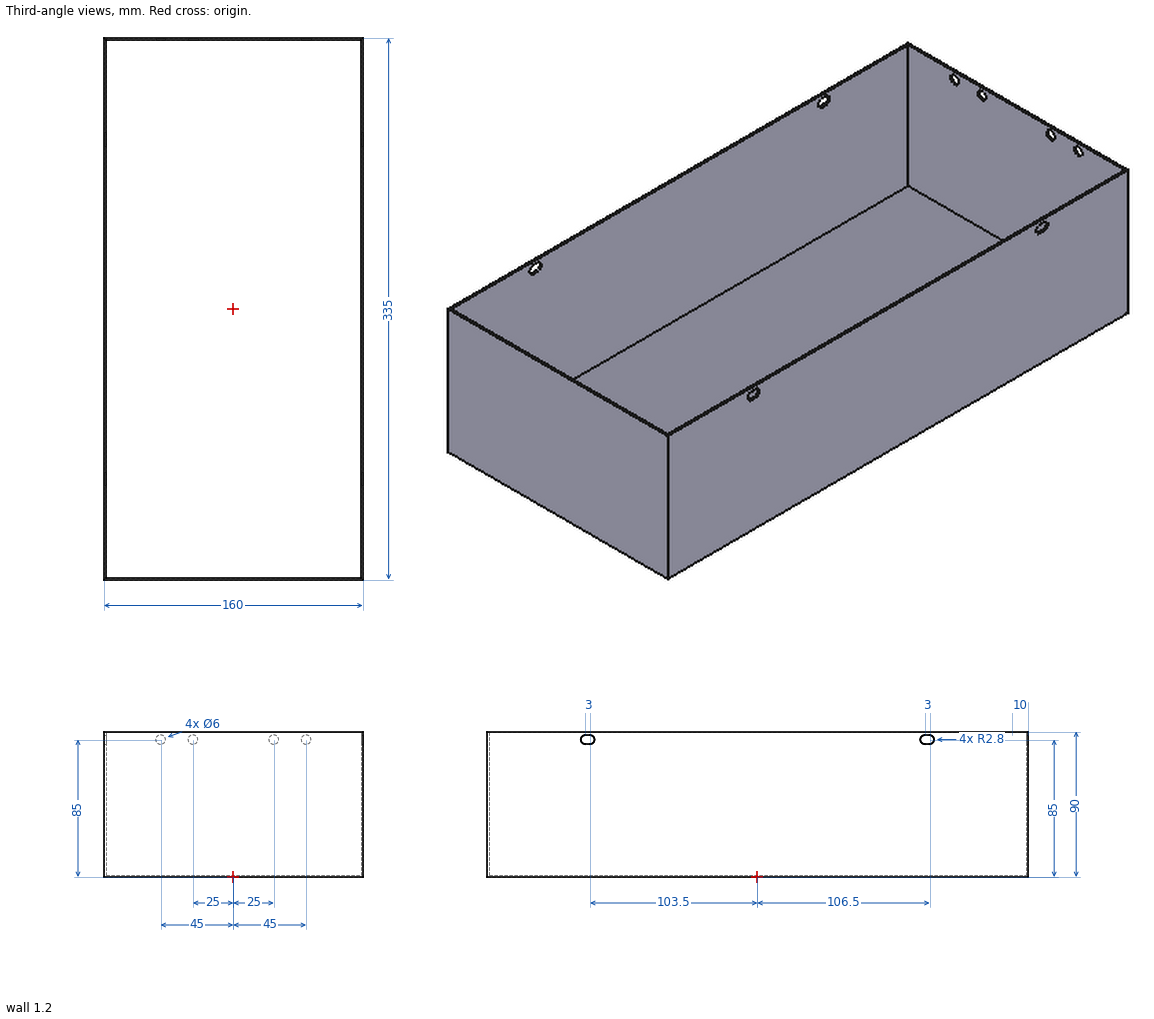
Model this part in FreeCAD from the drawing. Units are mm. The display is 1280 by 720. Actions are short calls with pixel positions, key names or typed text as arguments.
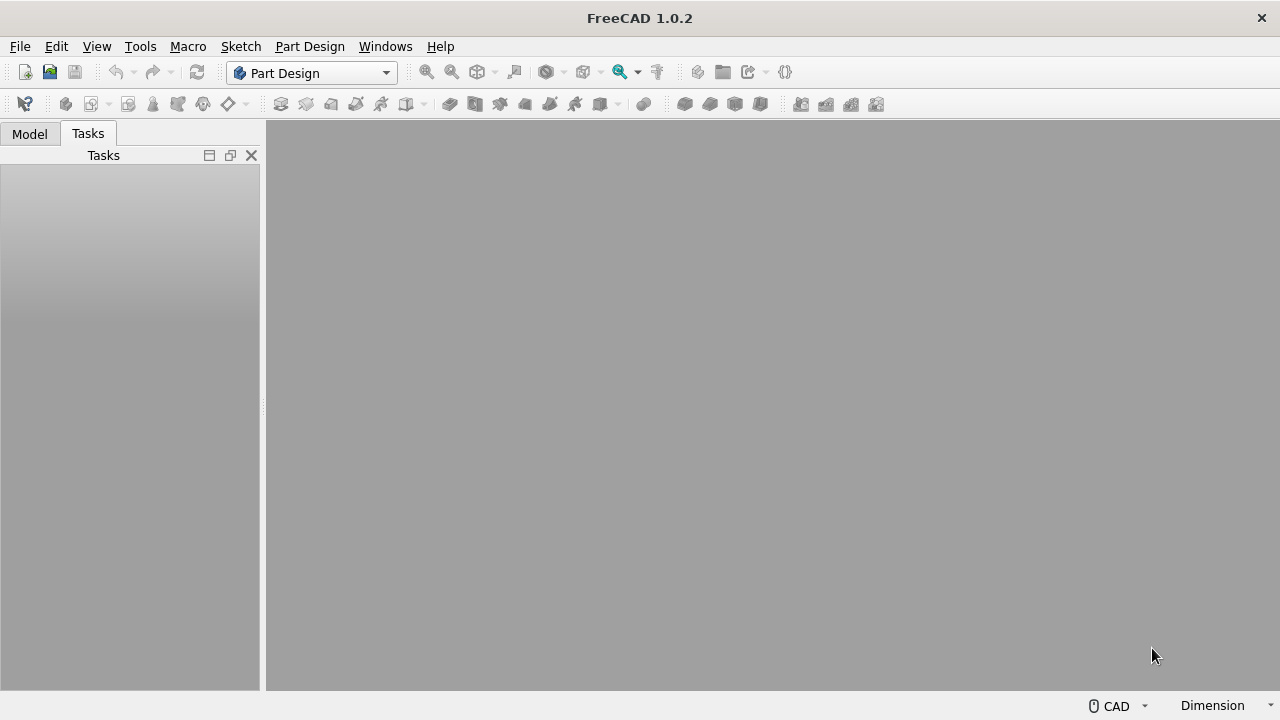
click(25, 72)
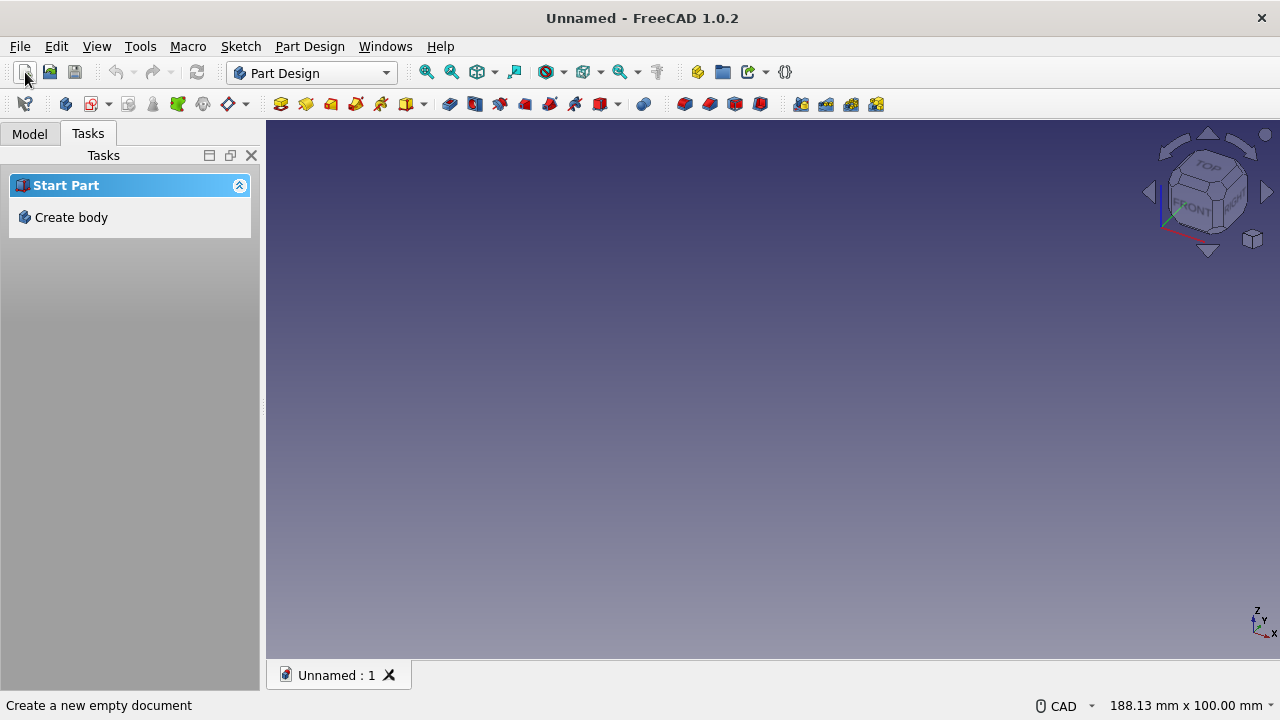
click(90, 104)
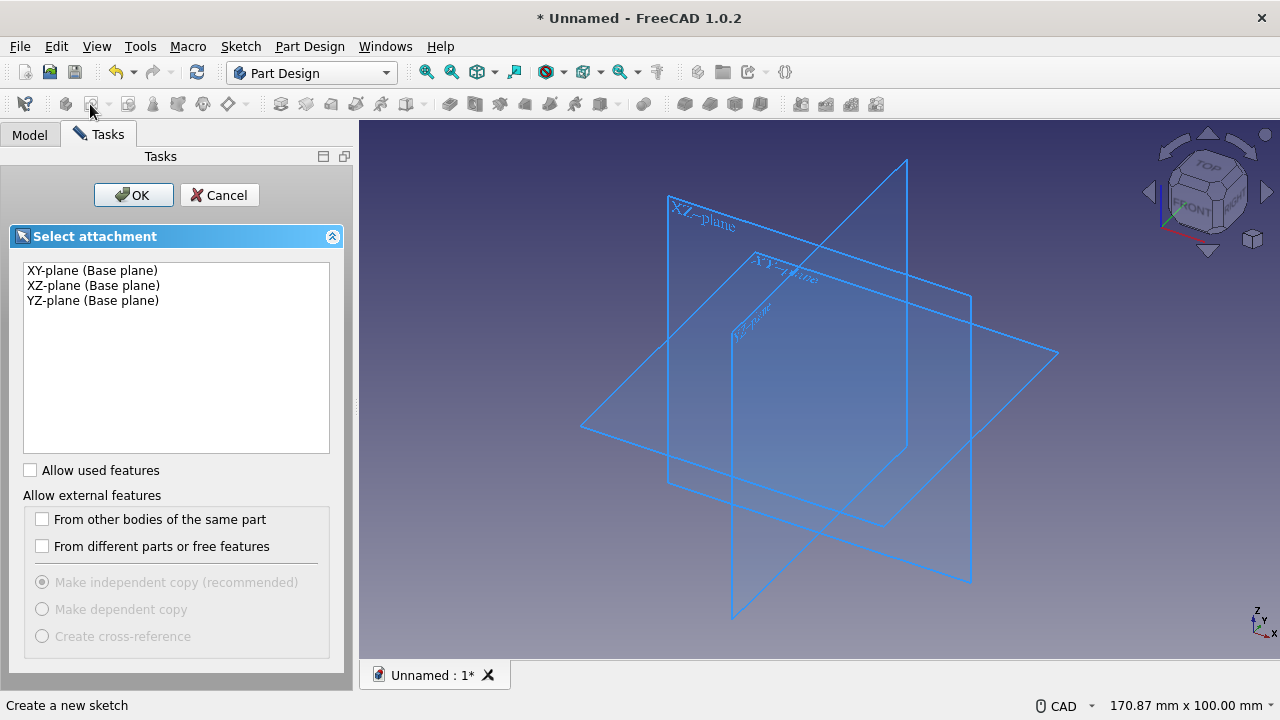
click(84, 270)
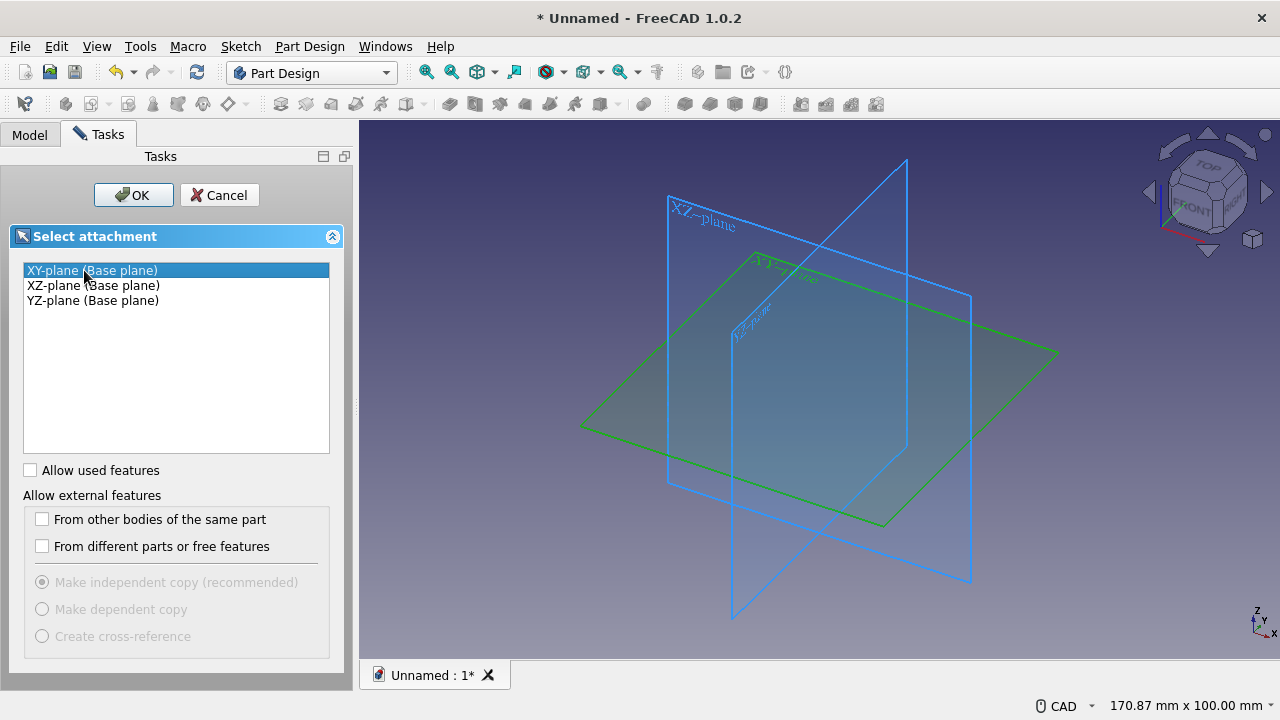
click(134, 195)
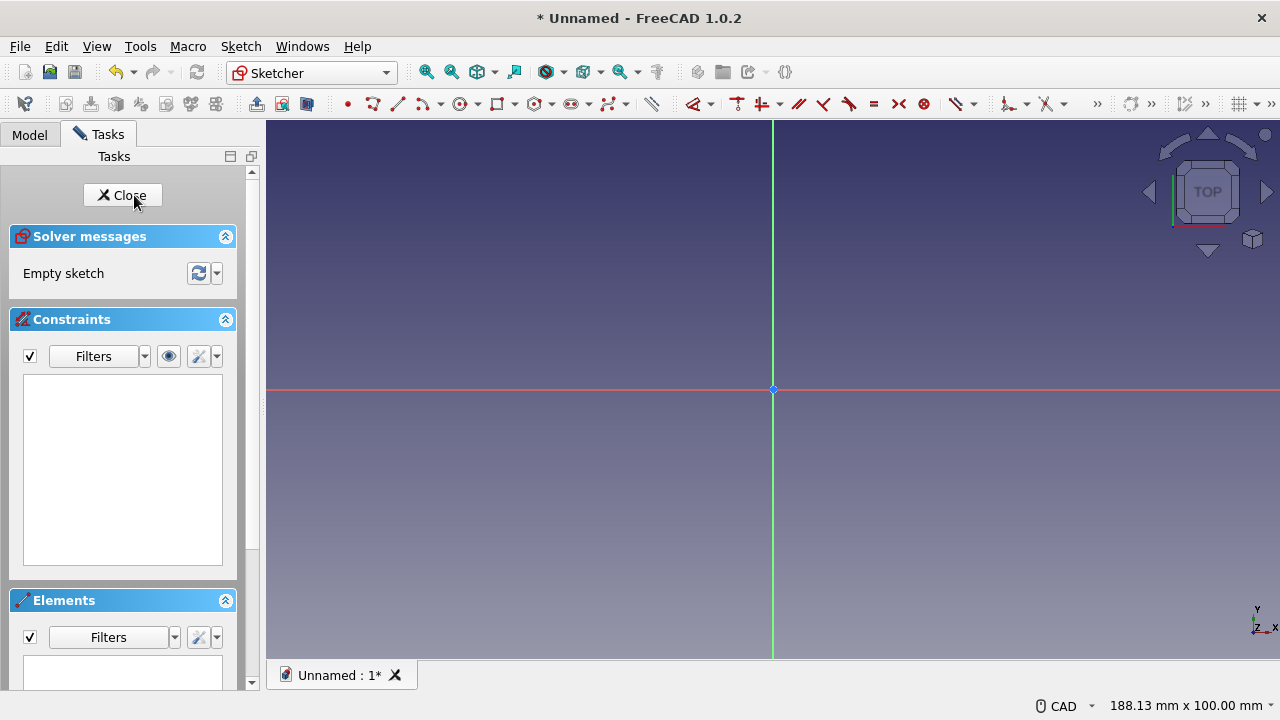
scroll(687, 389, down, 8)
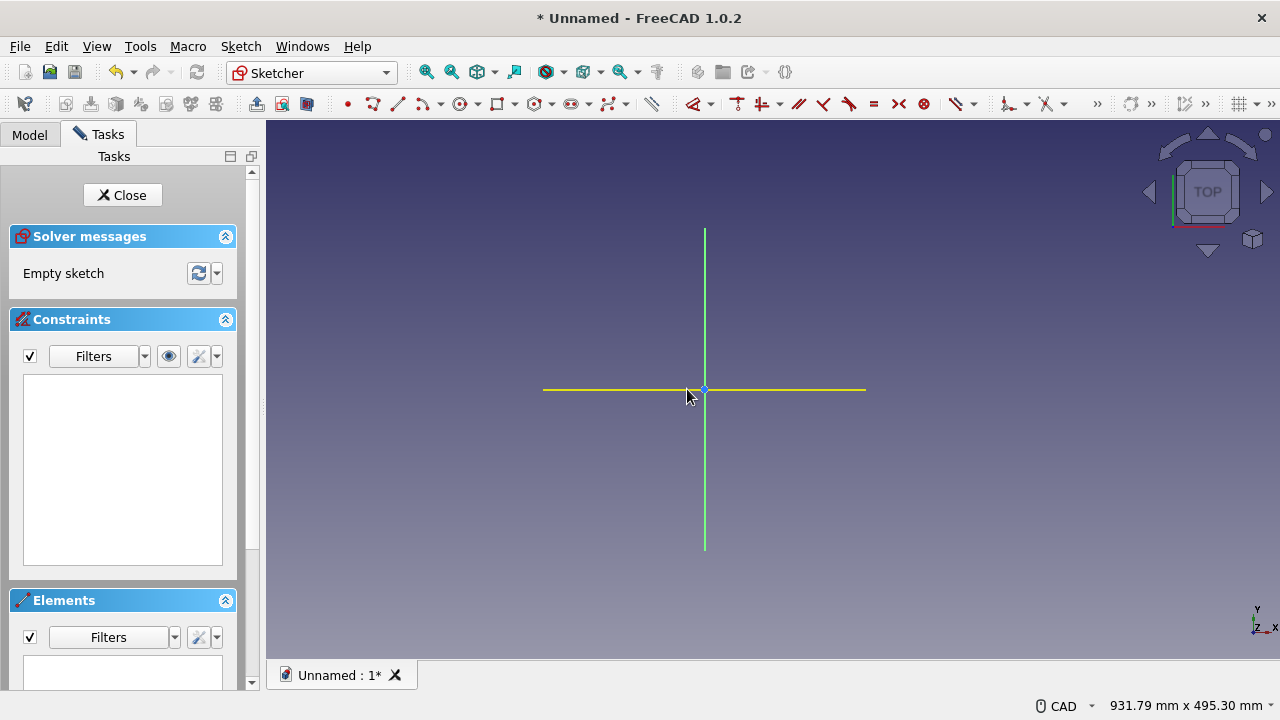
key(g)
key(v)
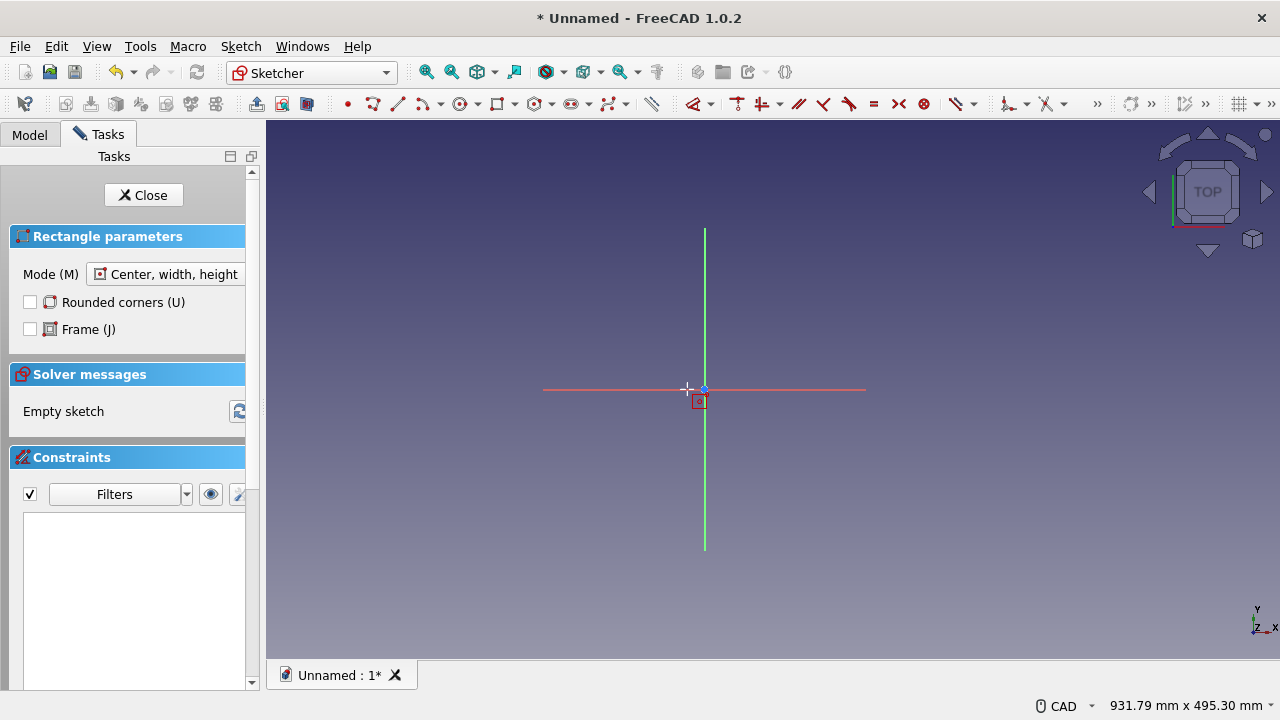
click(705, 390)
click(792, 207)
key(Escape)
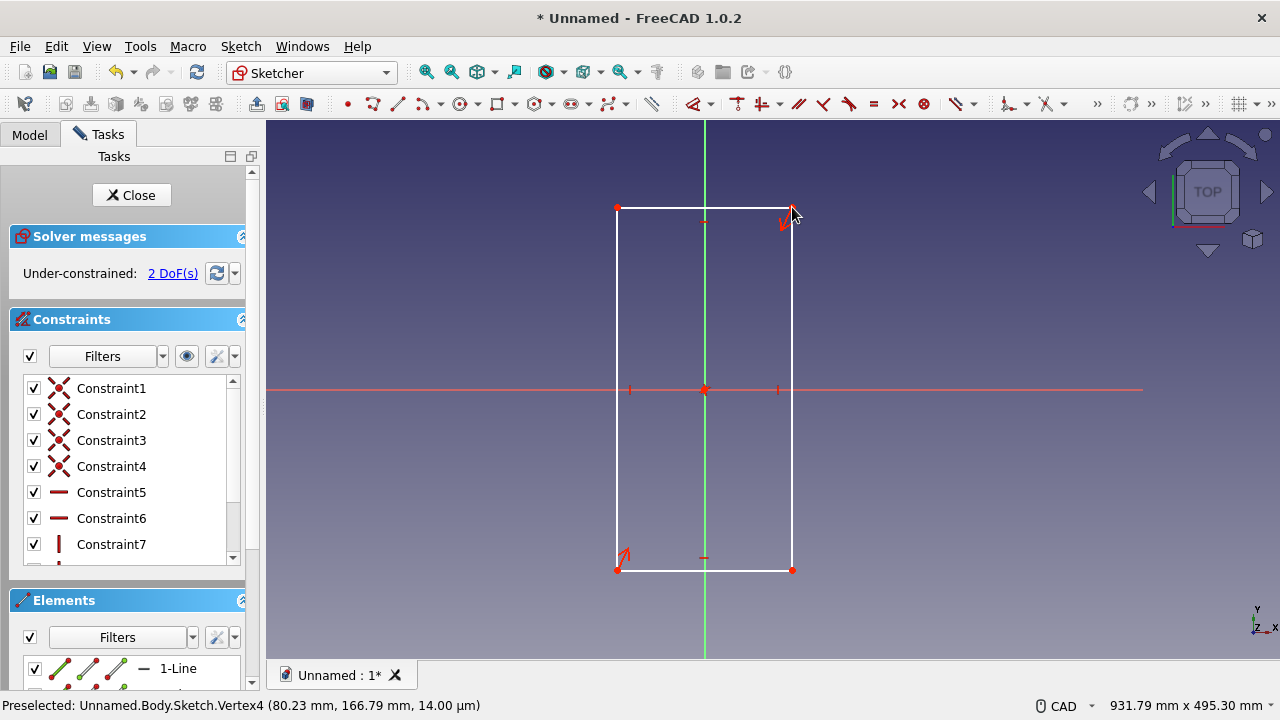
click(692, 104)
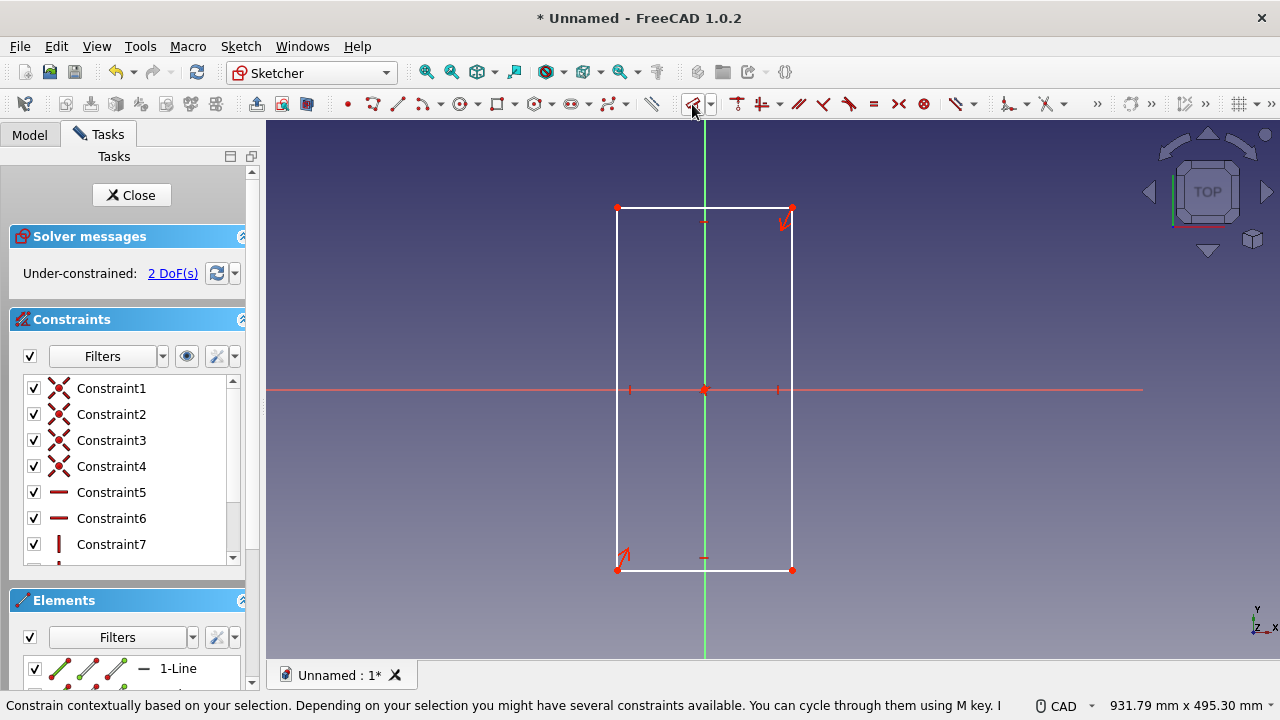
click(670, 571)
click(665, 605)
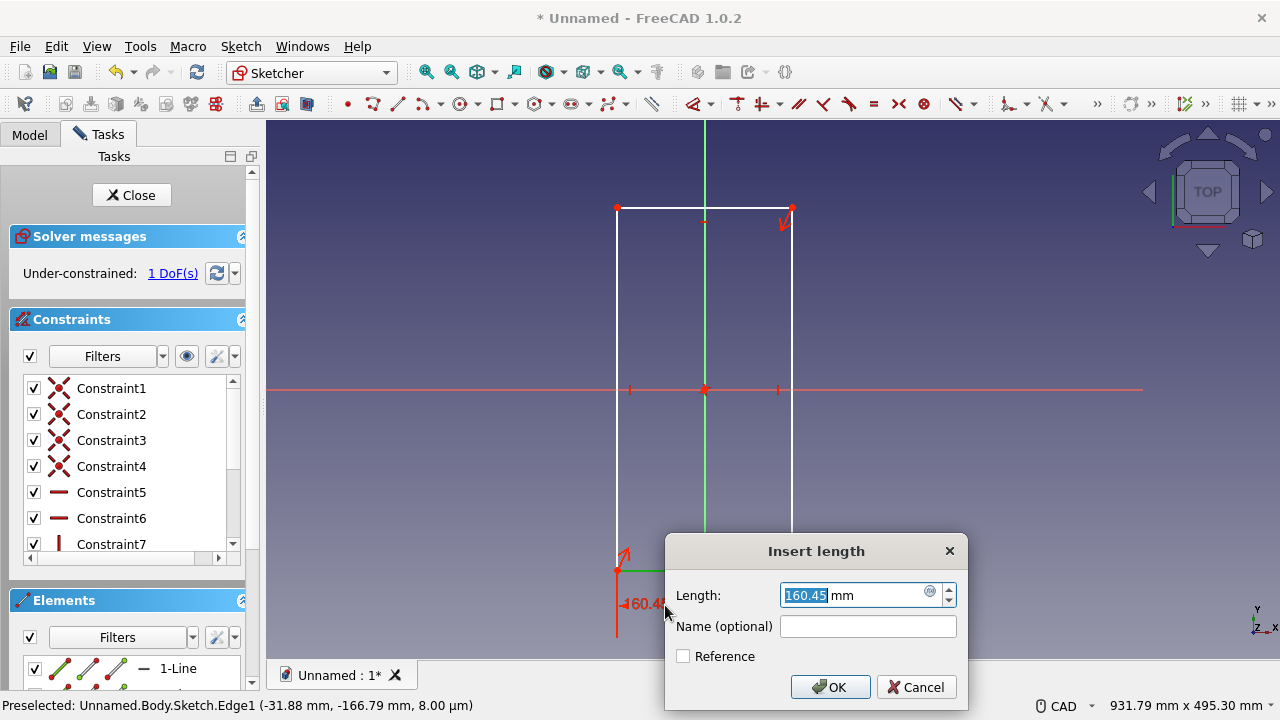
text(160)
key(Return)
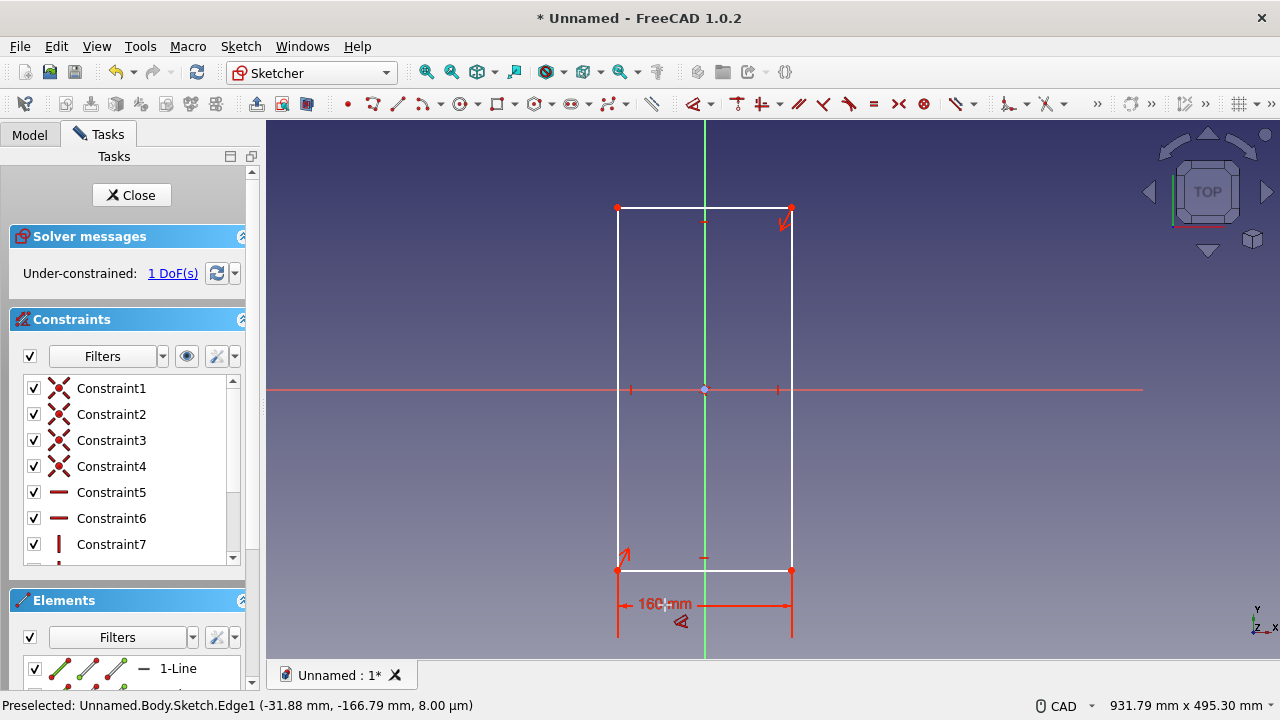
click(792, 462)
click(826, 306)